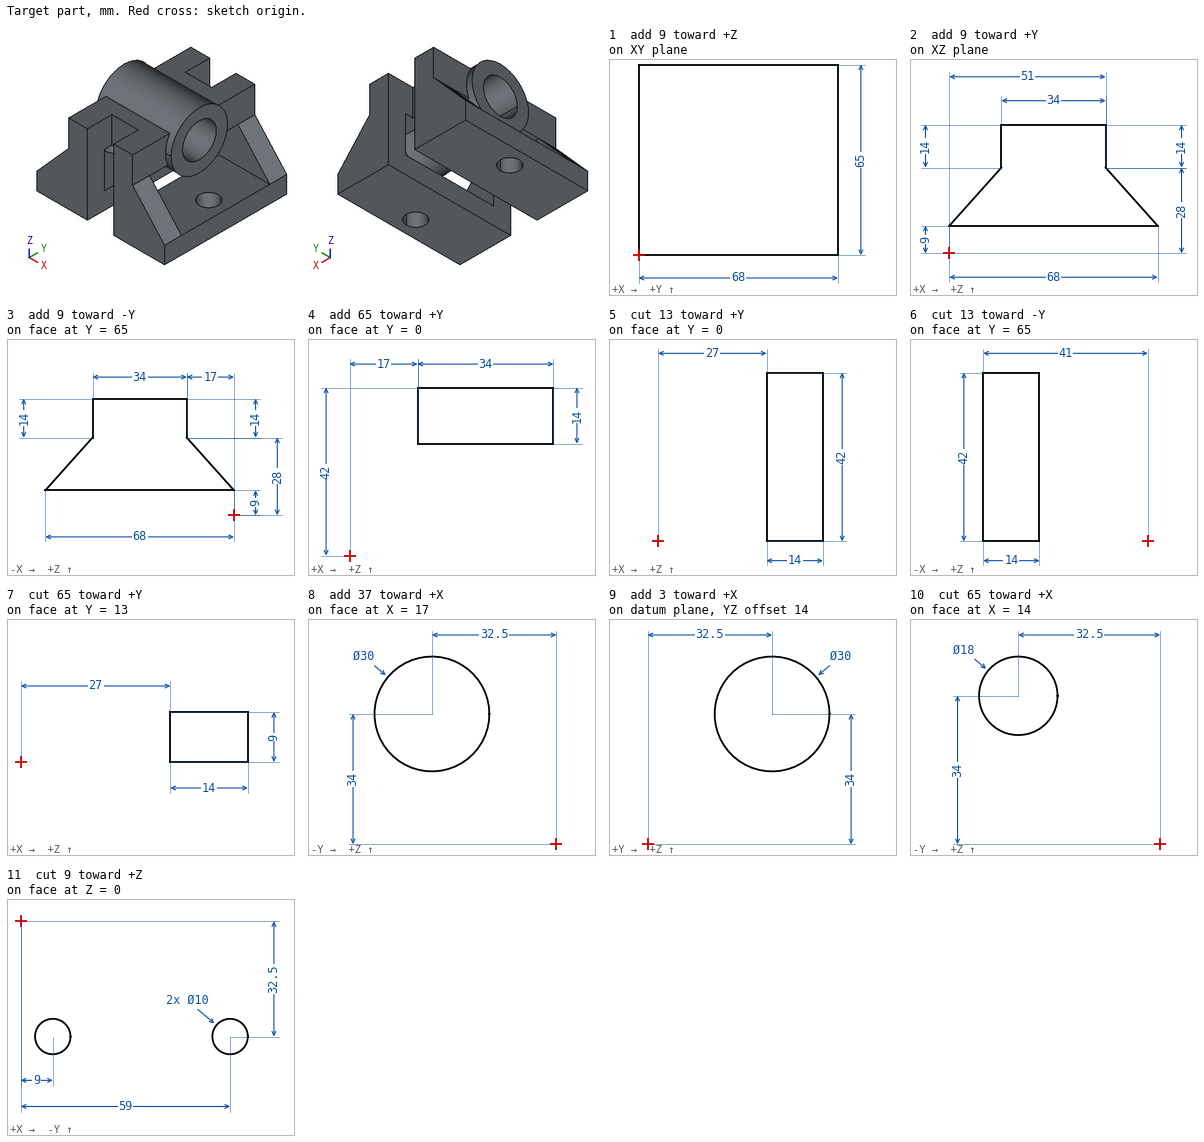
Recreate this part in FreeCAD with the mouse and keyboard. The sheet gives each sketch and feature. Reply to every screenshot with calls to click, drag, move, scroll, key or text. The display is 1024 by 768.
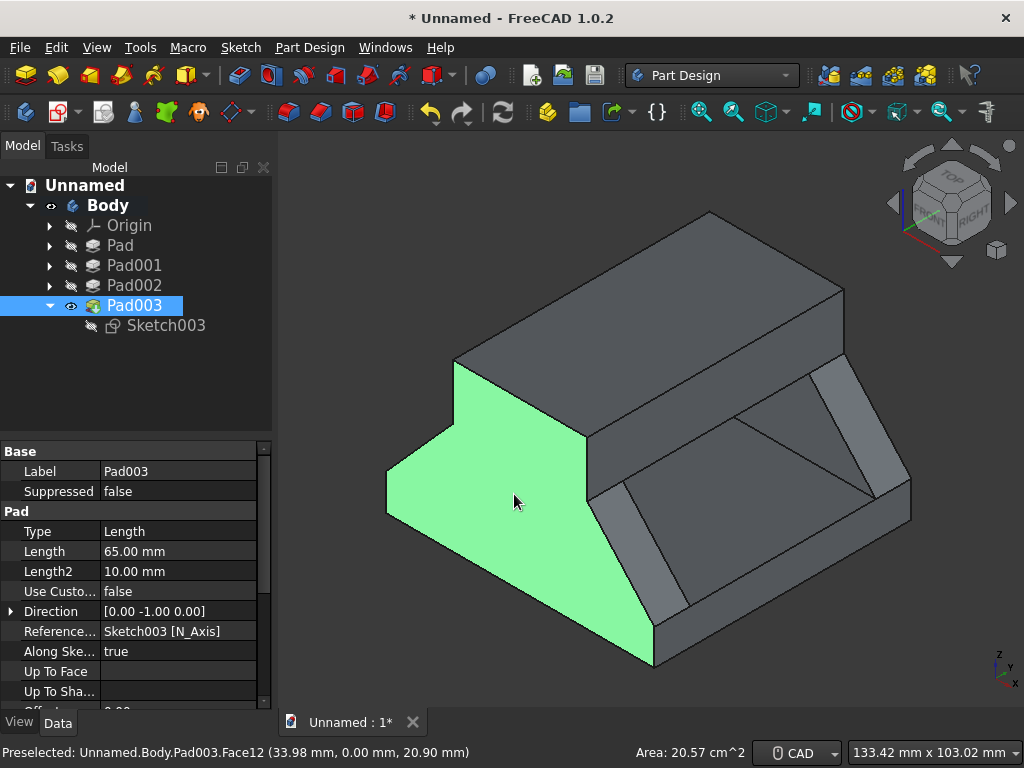
click(58, 112)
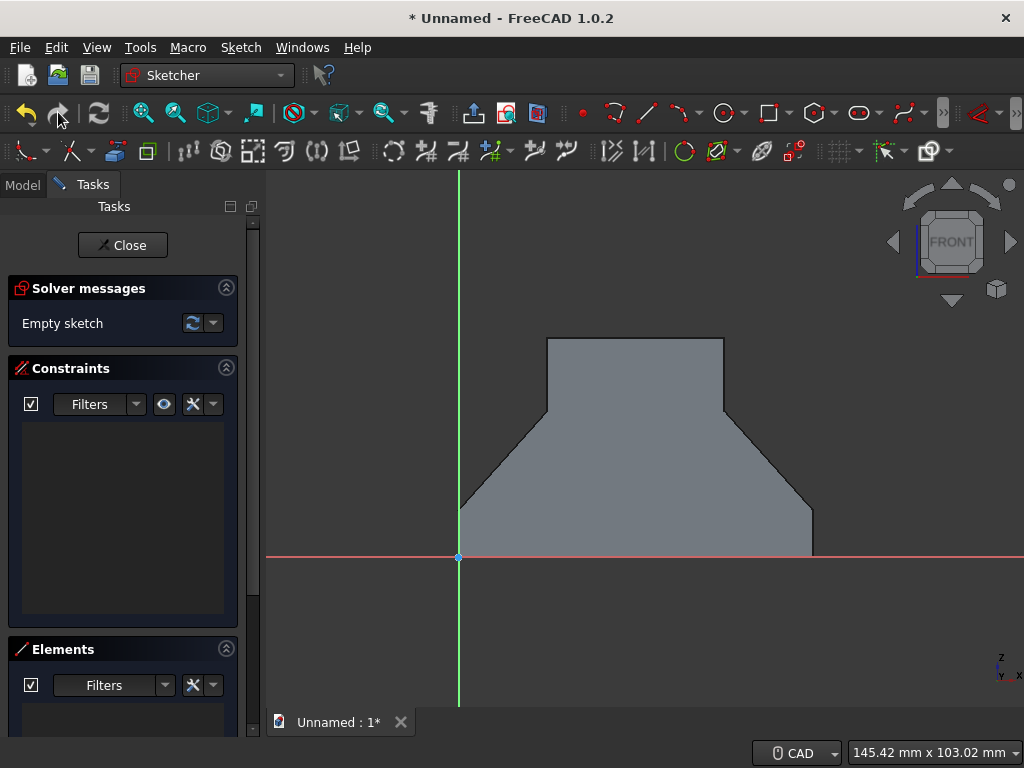
scroll(543, 466, up, 2)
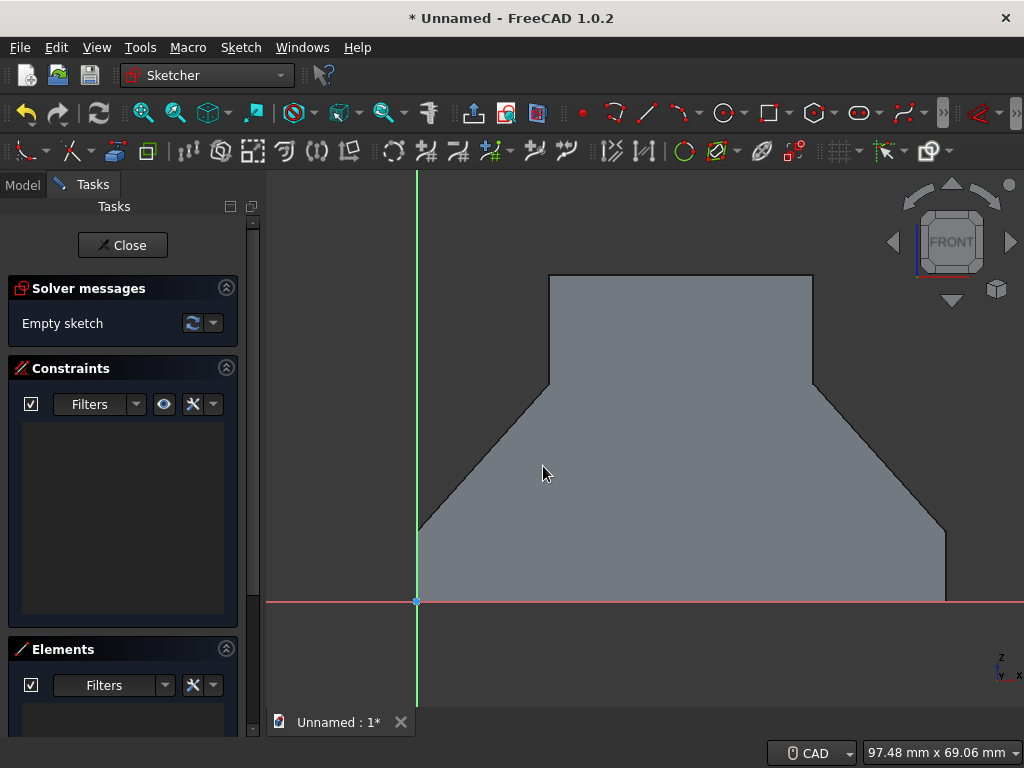
click(770, 114)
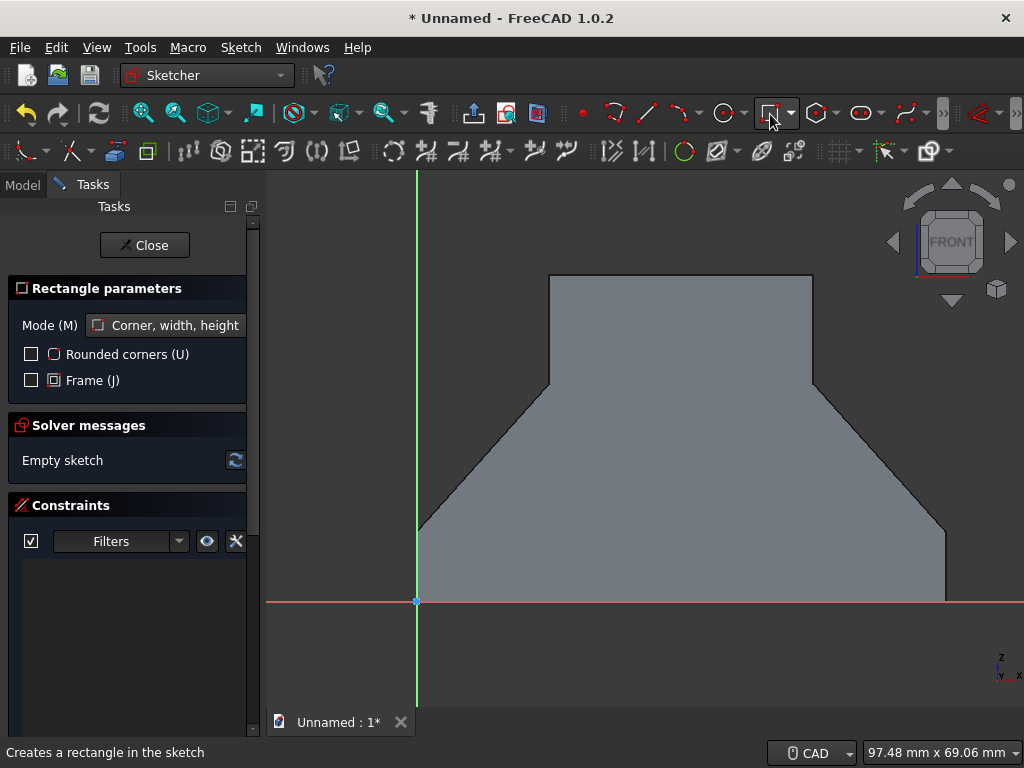
click(627, 275)
click(736, 602)
key(Escape)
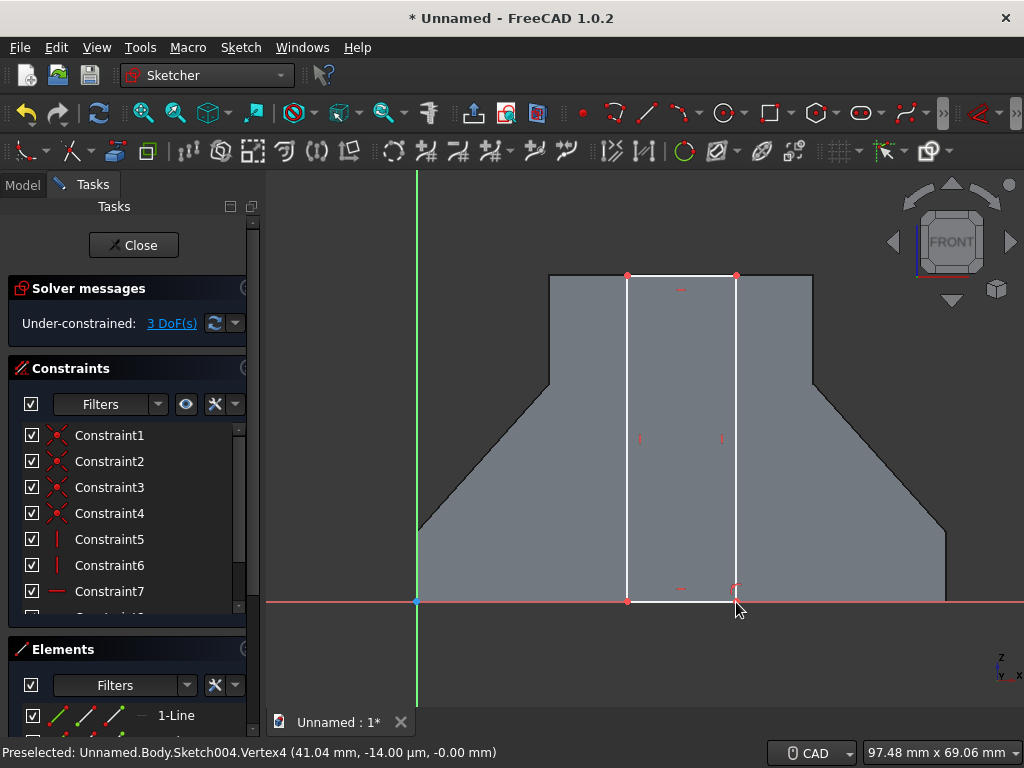
key(d)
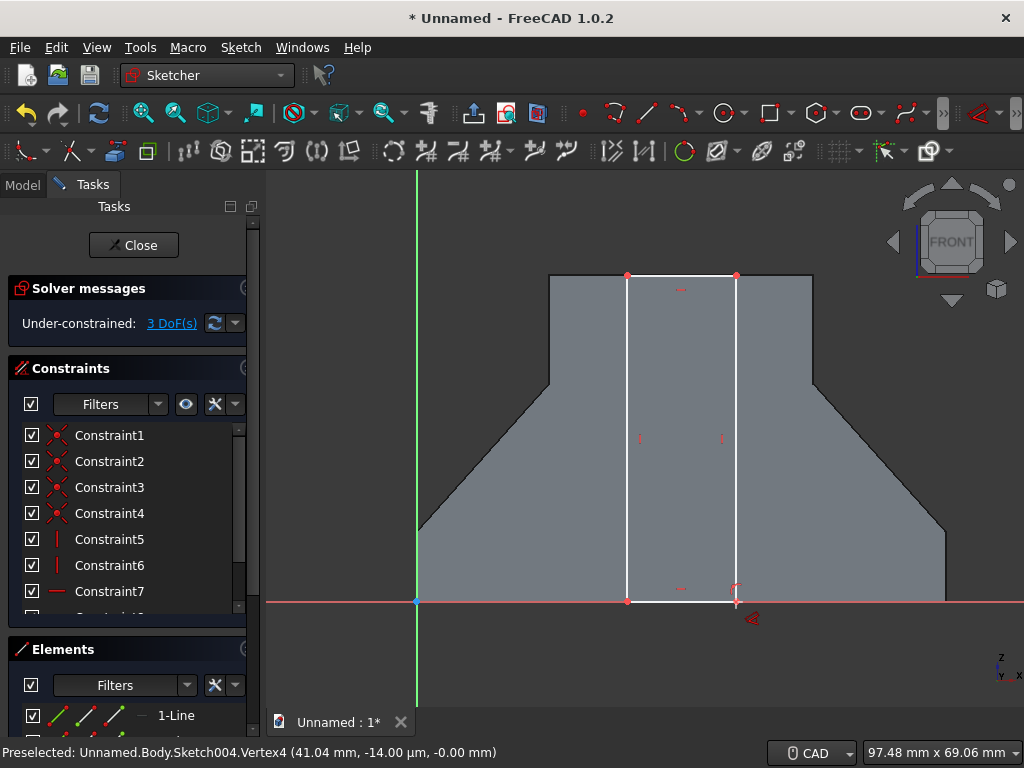
click(627, 374)
click(661, 439)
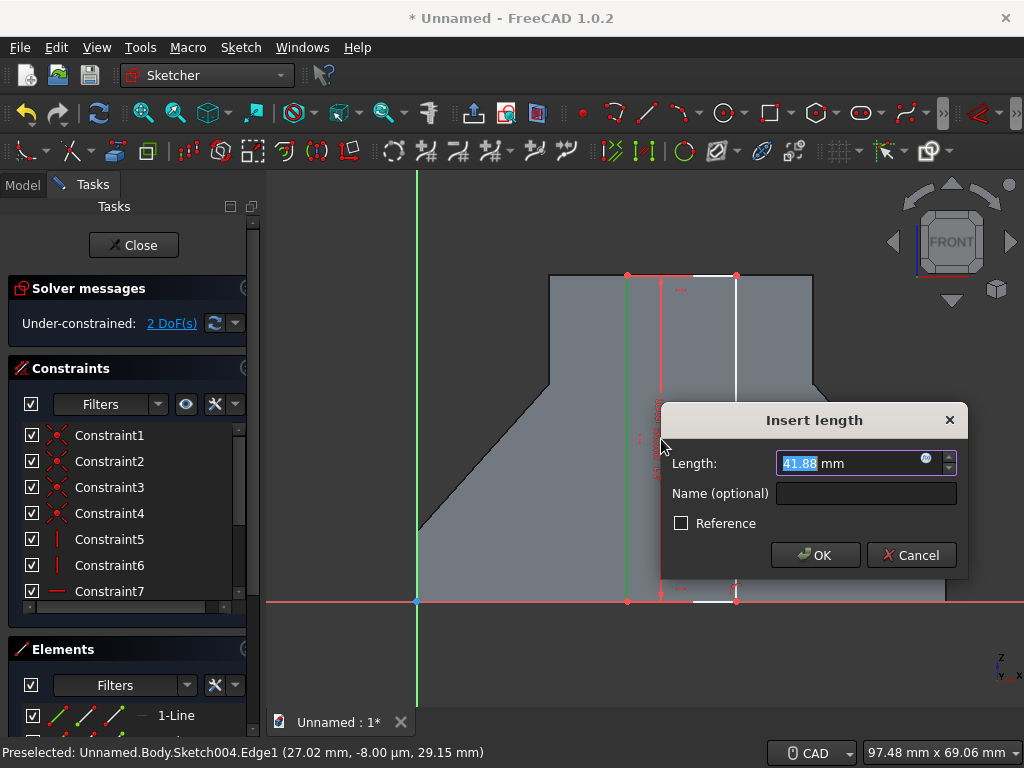
text(42)
key(Return)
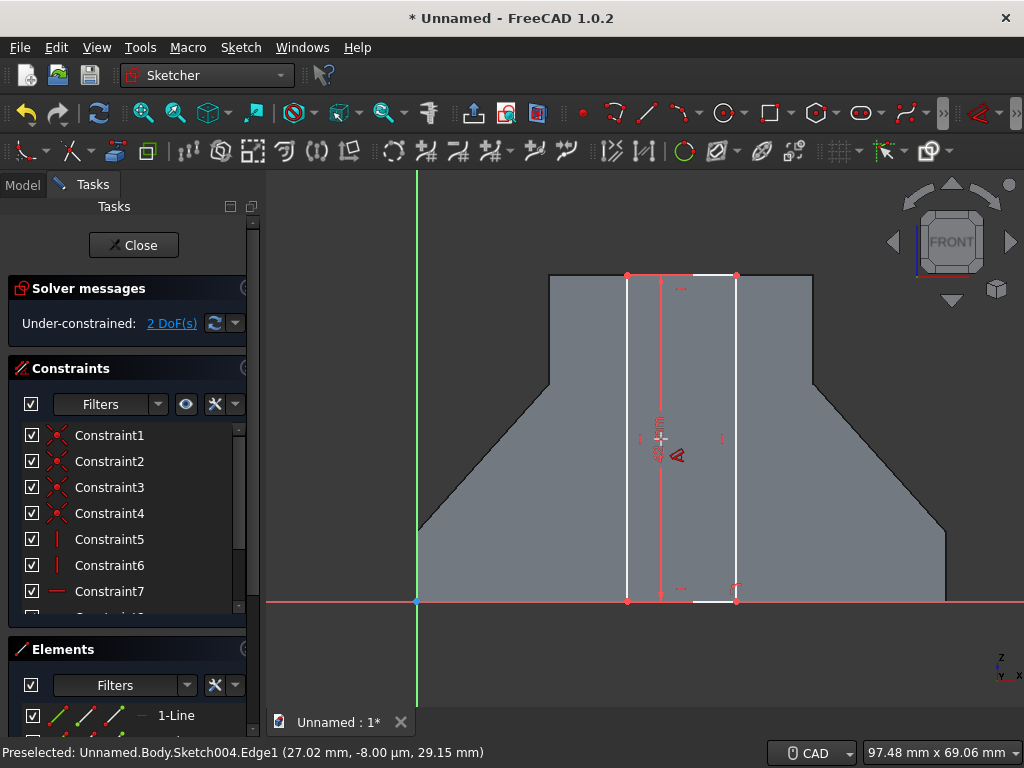
click(660, 602)
click(681, 636)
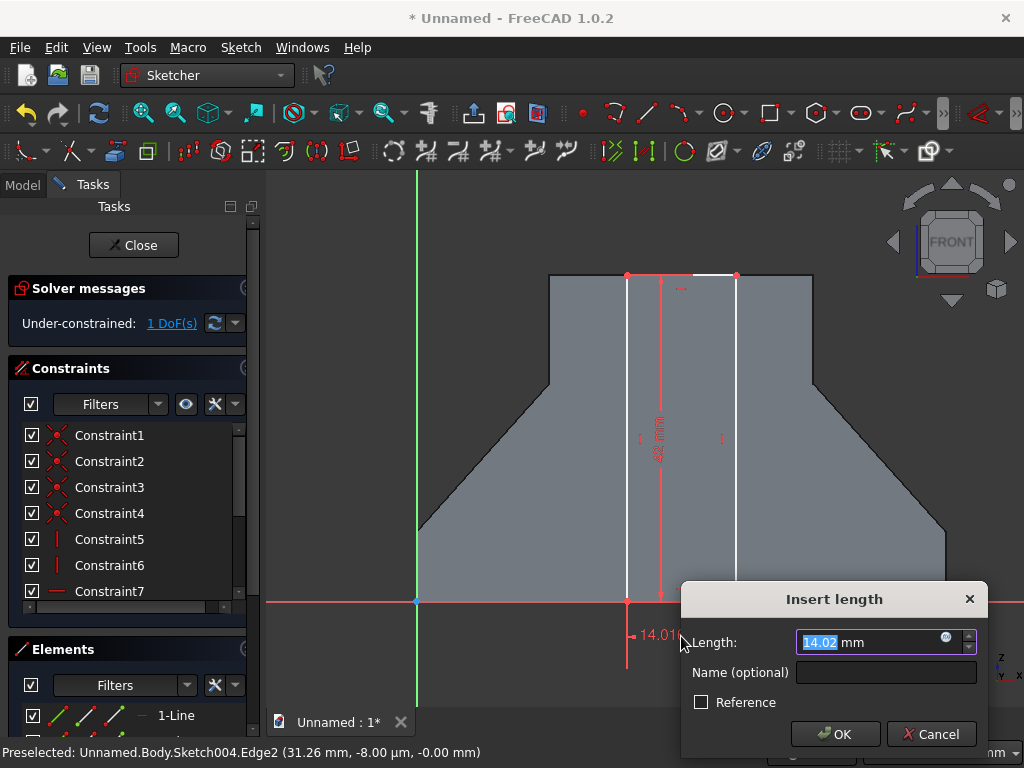
text(14)
key(Return)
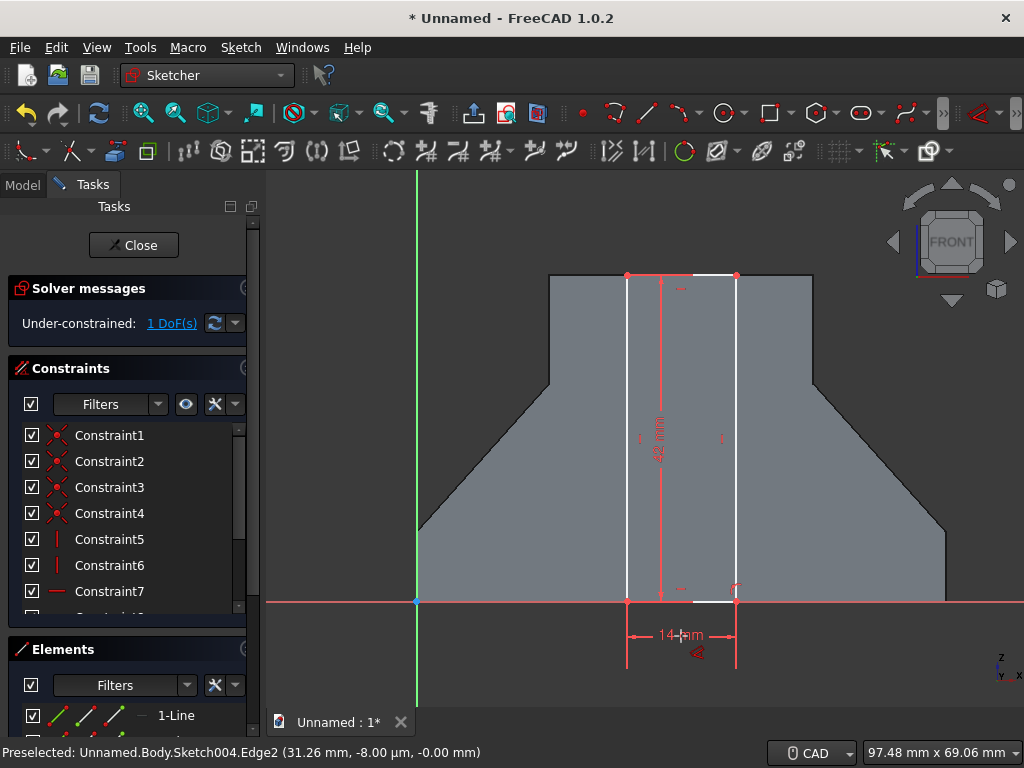
click(627, 275)
click(522, 636)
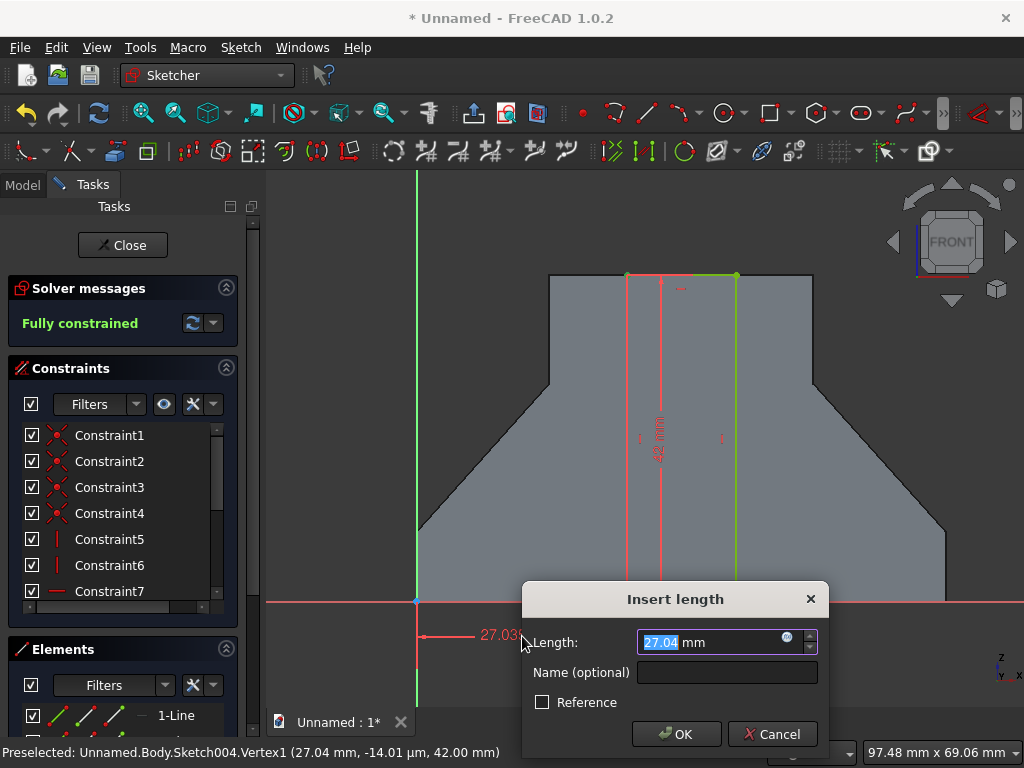
text(27)
key(Return)
key(Escape)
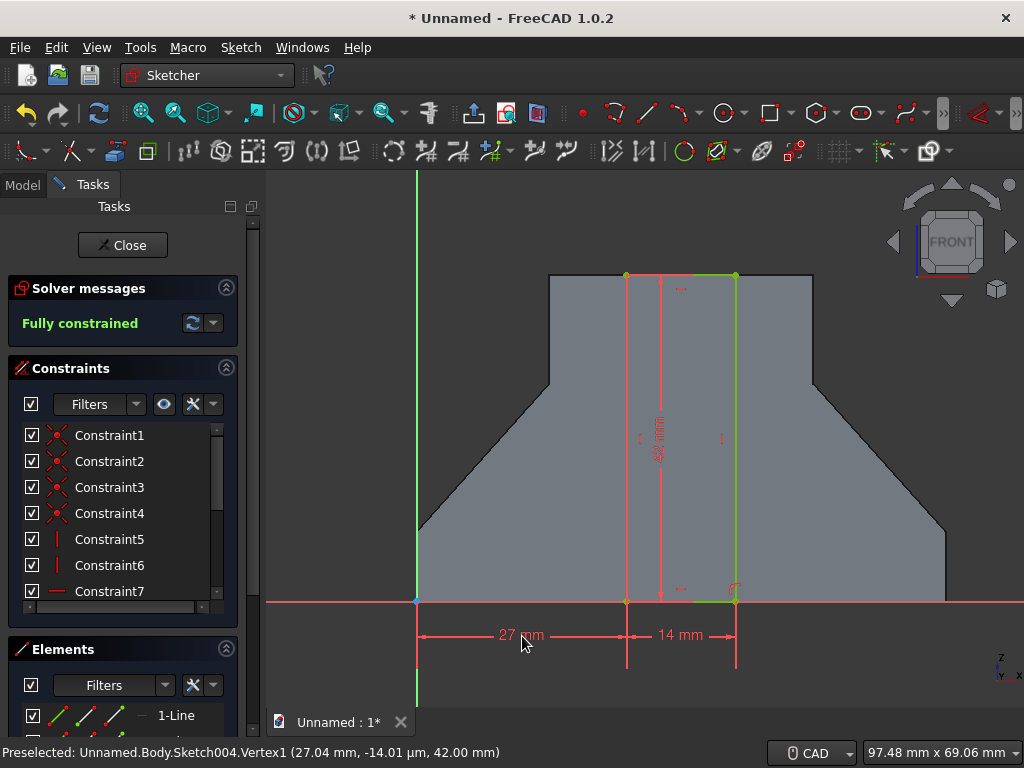
click(123, 245)